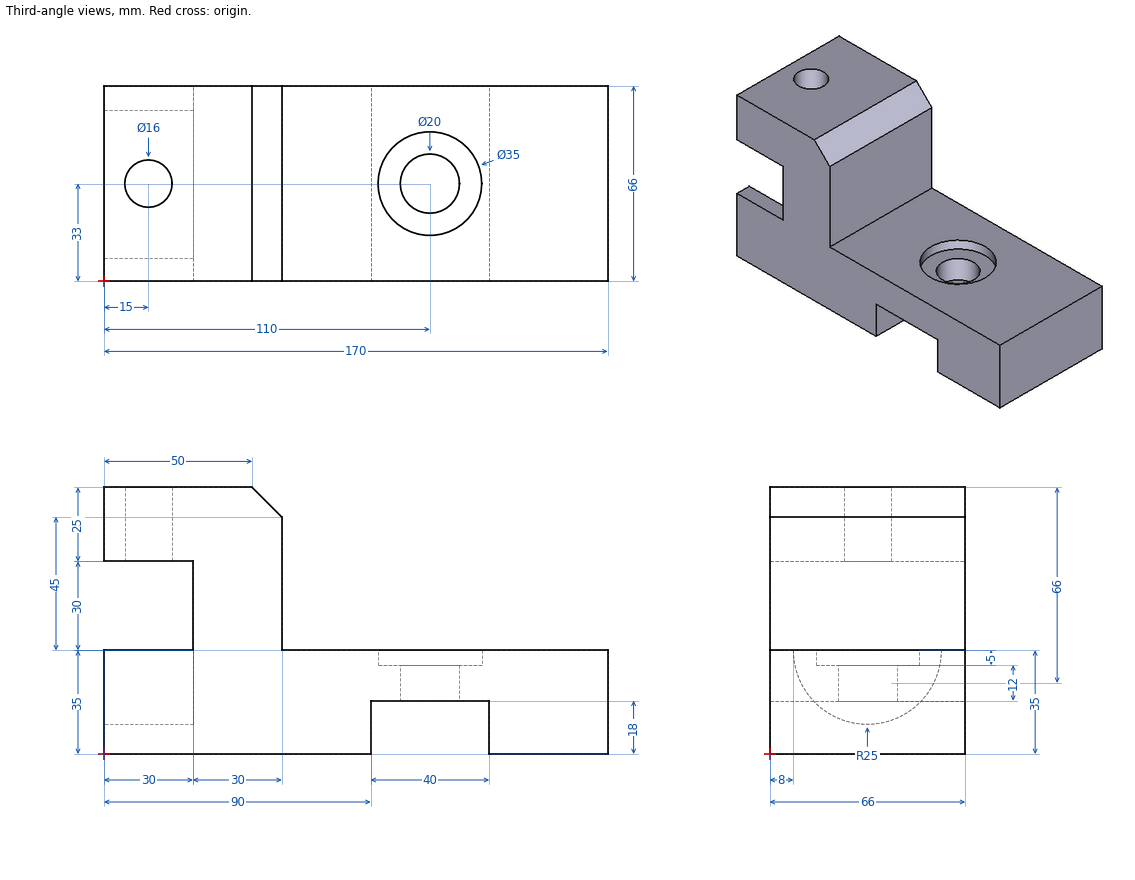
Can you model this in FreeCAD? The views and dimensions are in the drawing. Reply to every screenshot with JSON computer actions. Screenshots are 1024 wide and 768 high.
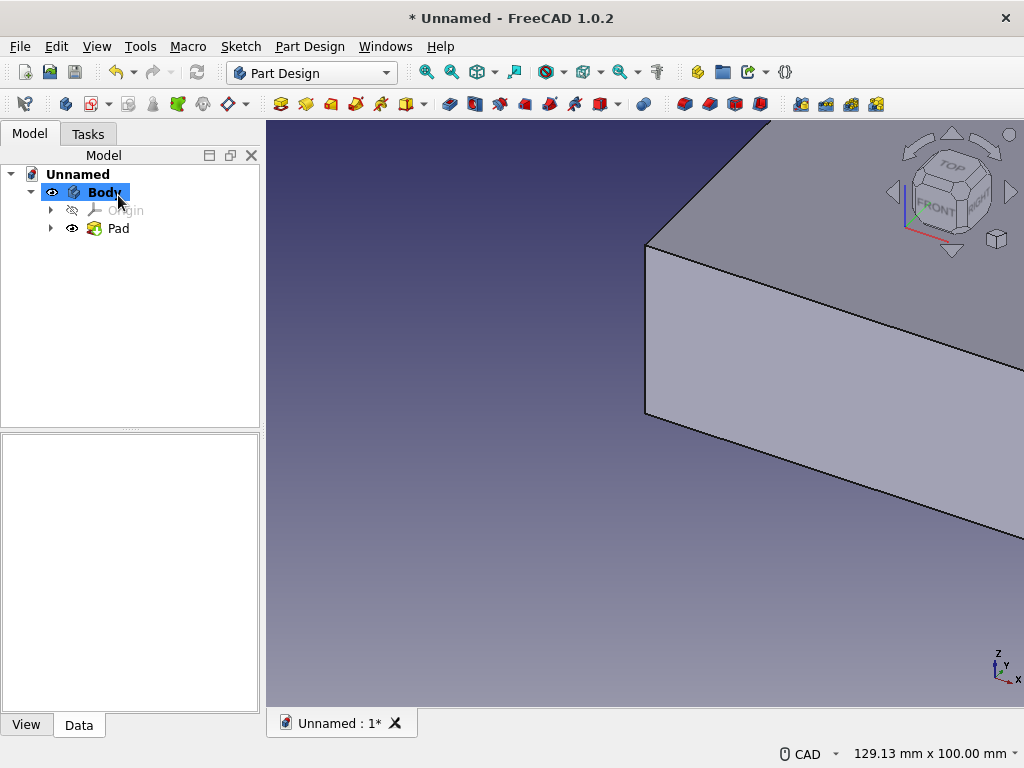
{"action": "key", "text": "v f"}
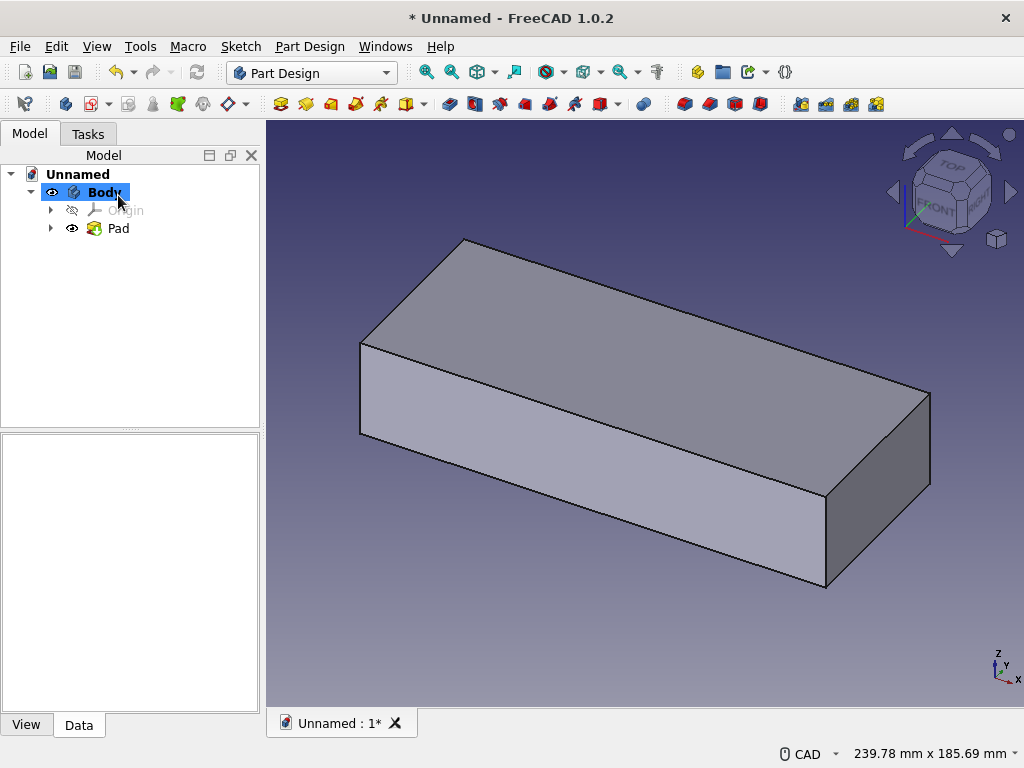
{"action": "left_click", "coordinate": [90, 104]}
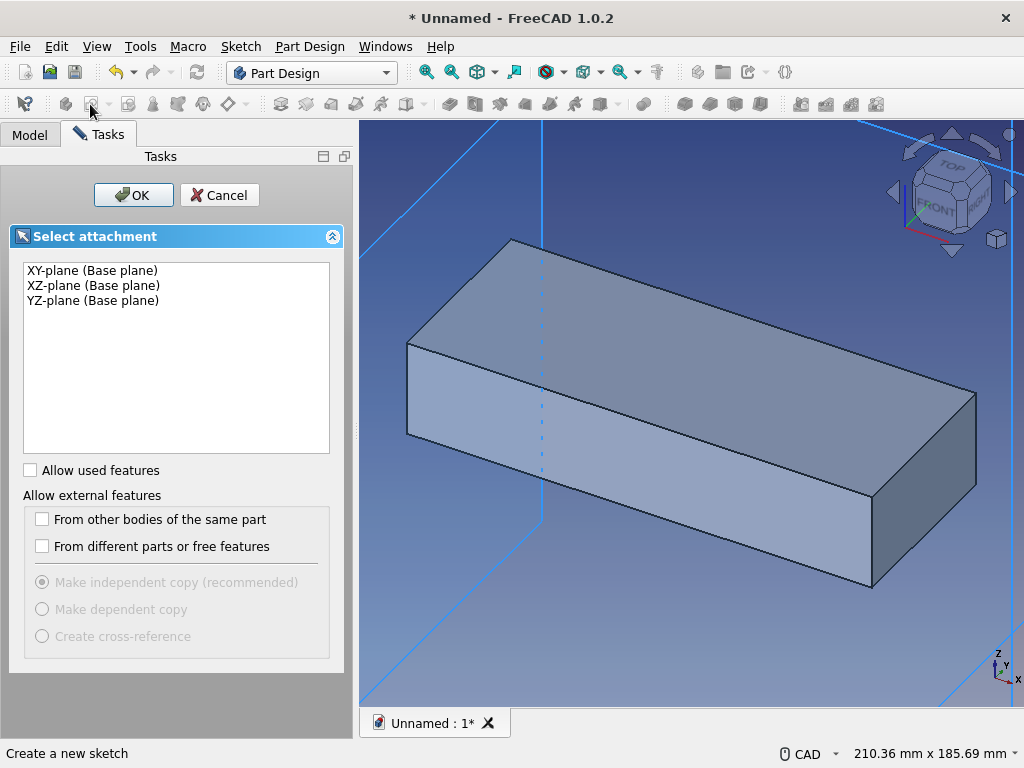
{"action": "left_click", "coordinate": [84, 286]}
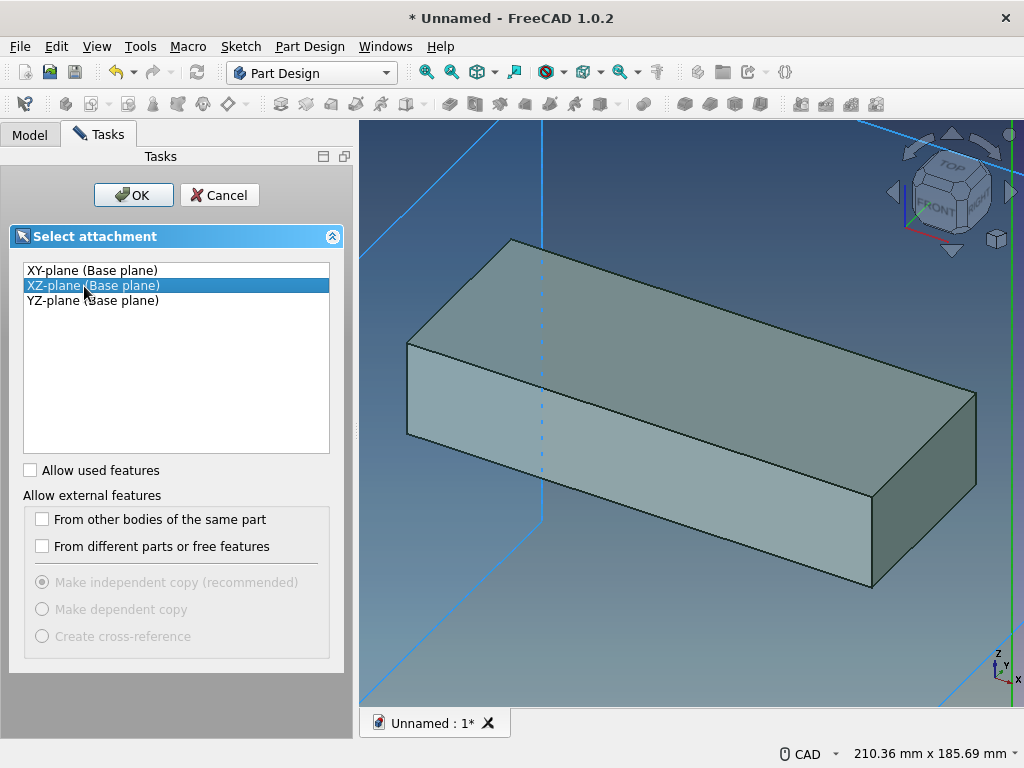
{"action": "left_click", "coordinate": [134, 195]}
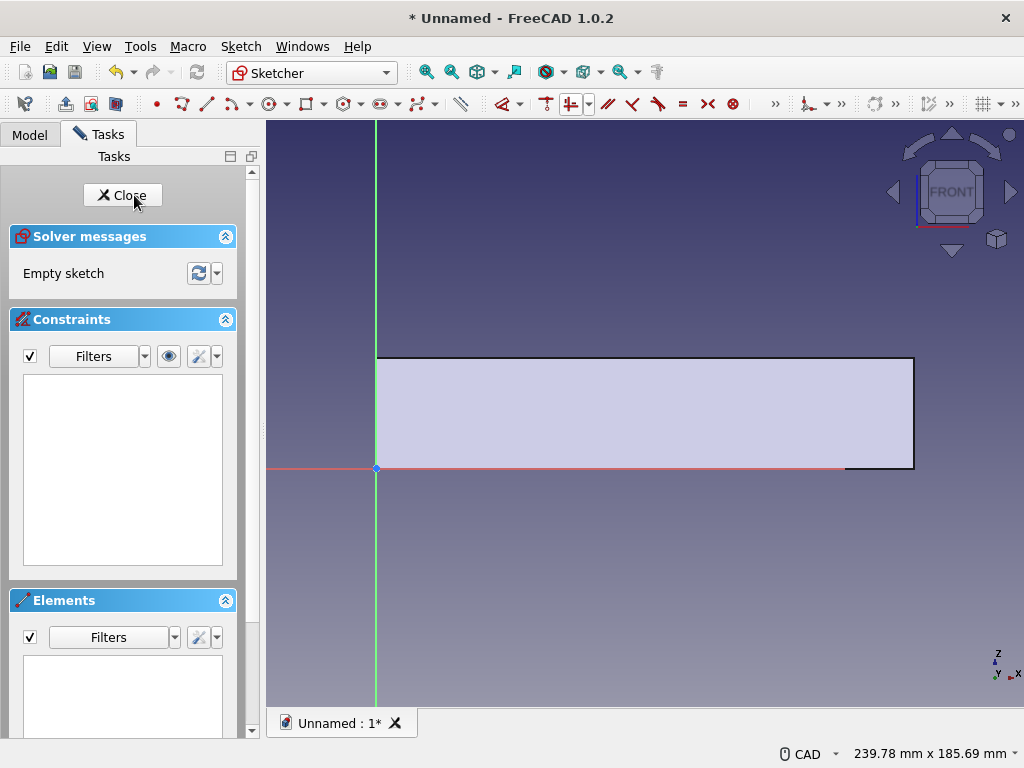
{"action": "scroll", "coordinate": [788, 452], "scroll_direction": "up", "scroll_amount": 6}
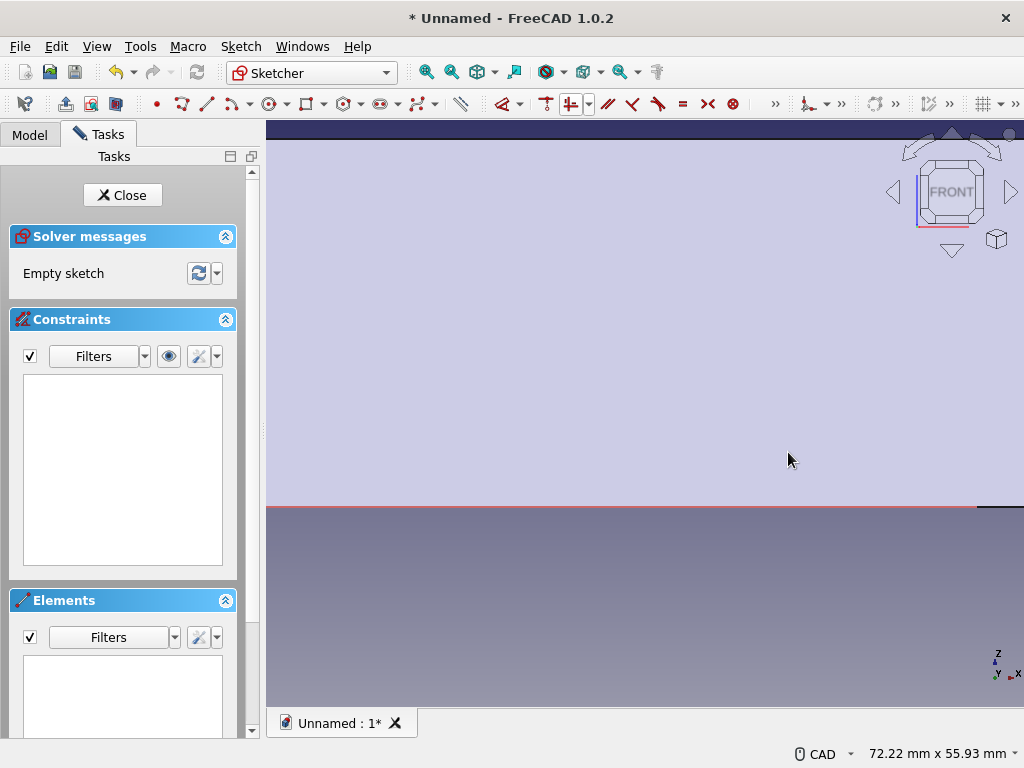
{"action": "left_click", "coordinate": [306, 104]}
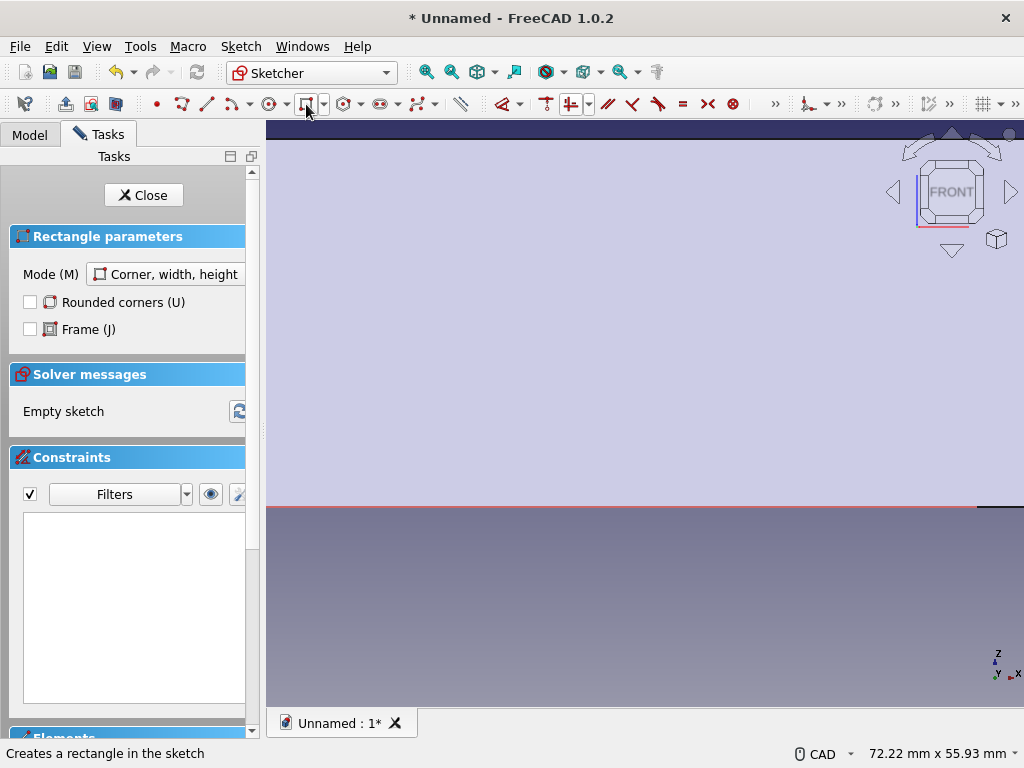
{"action": "left_click", "coordinate": [364, 318]}
{"action": "left_click", "coordinate": [784, 507]}
{"action": "key", "text": "Escape"}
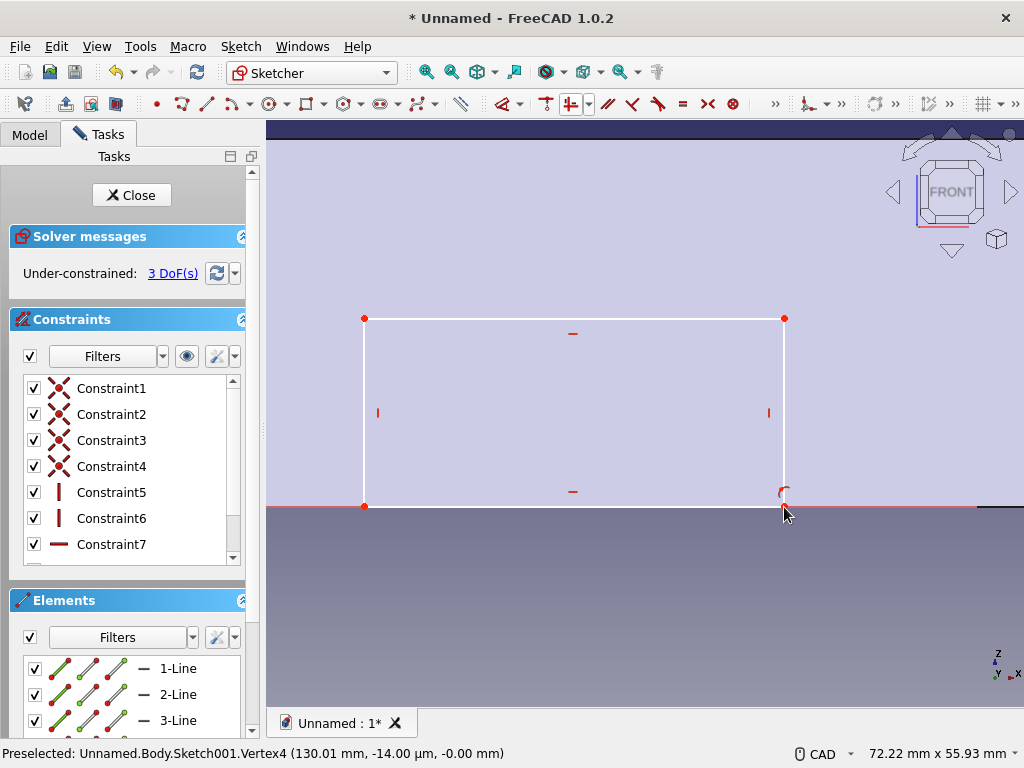
{"action": "left_click", "coordinate": [364, 375]}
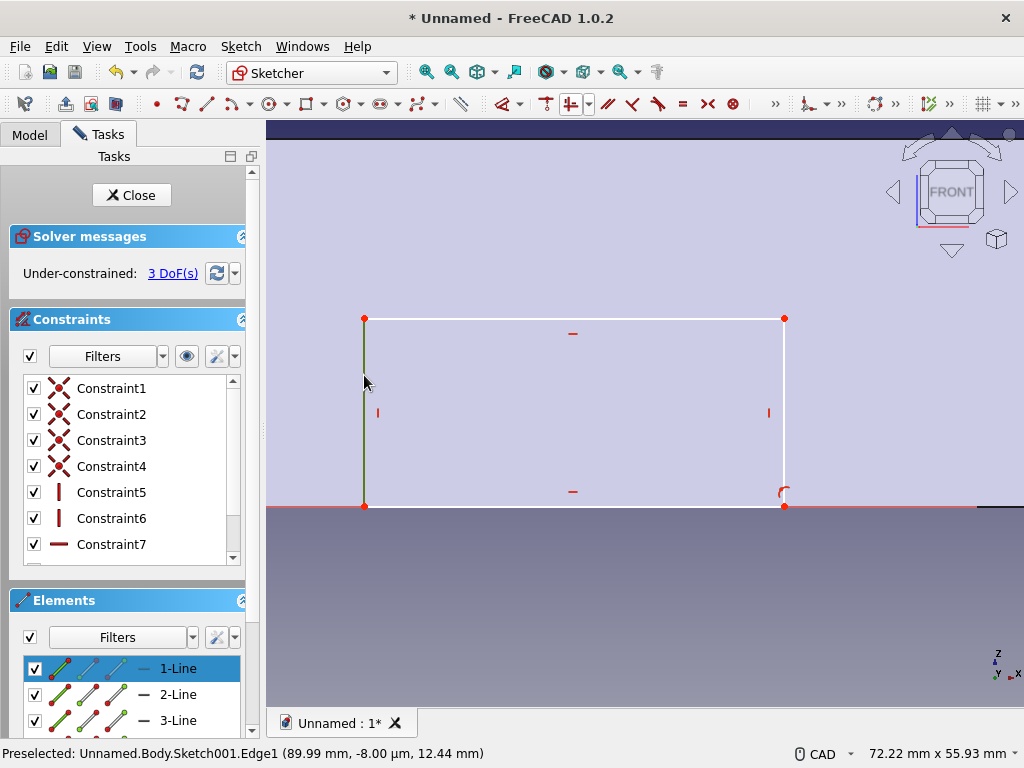
{"action": "left_click", "coordinate": [520, 104]}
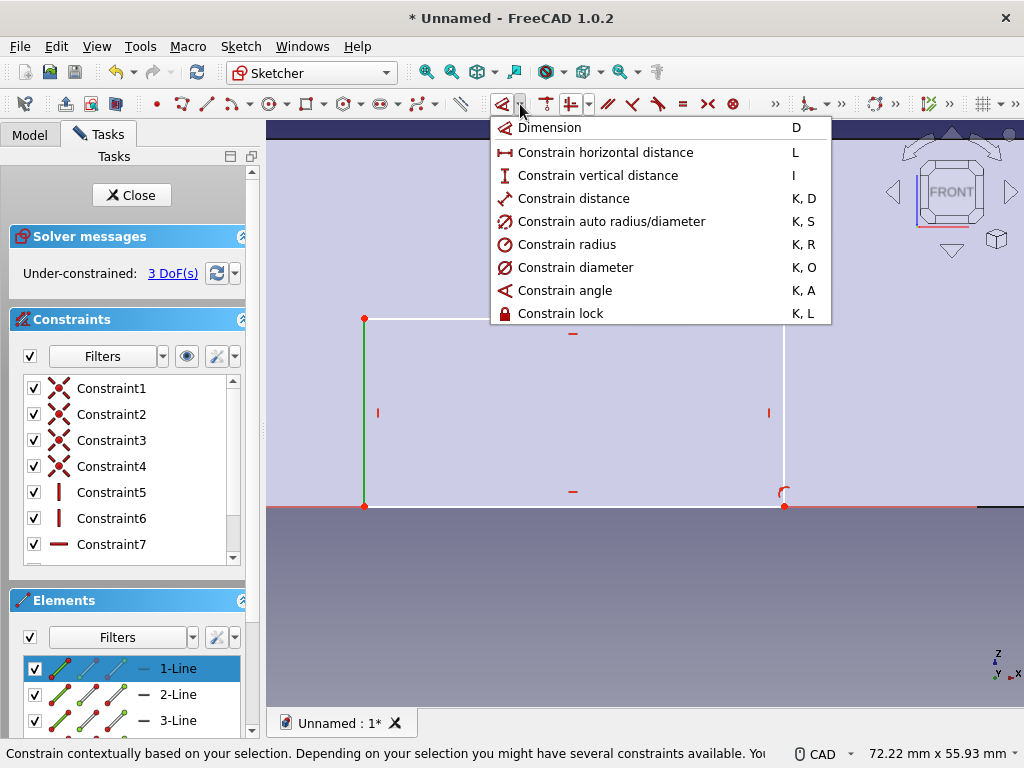
{"action": "left_click", "coordinate": [661, 176]}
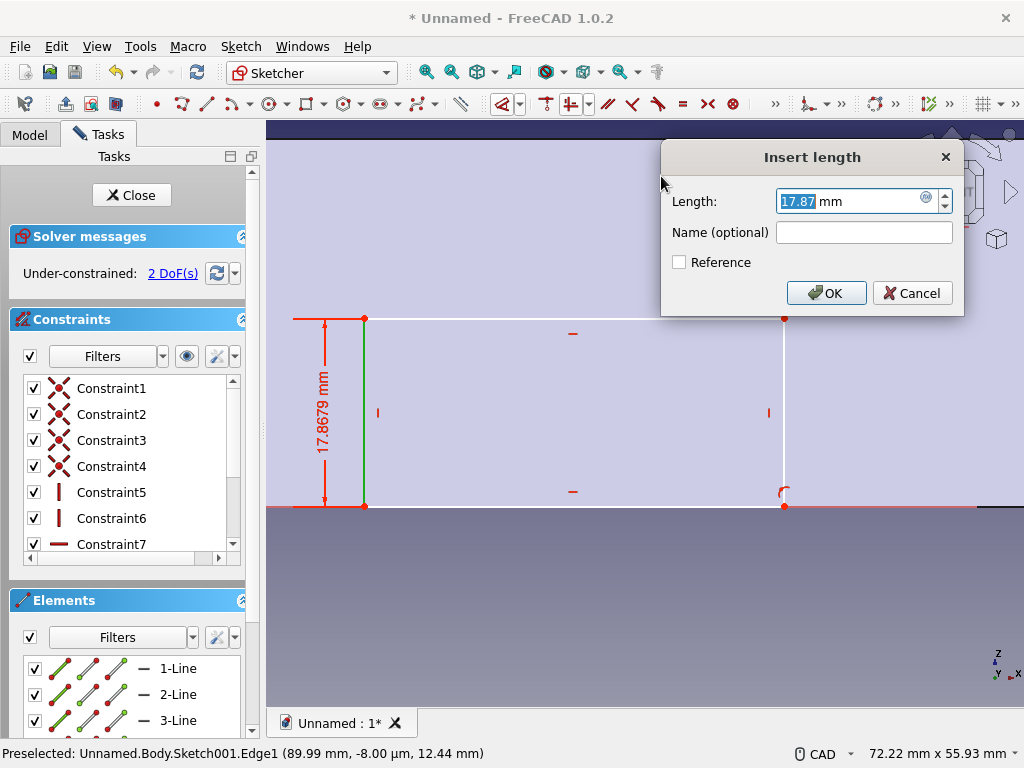
{"action": "type", "text": "18"}
{"action": "key", "text": "Return"}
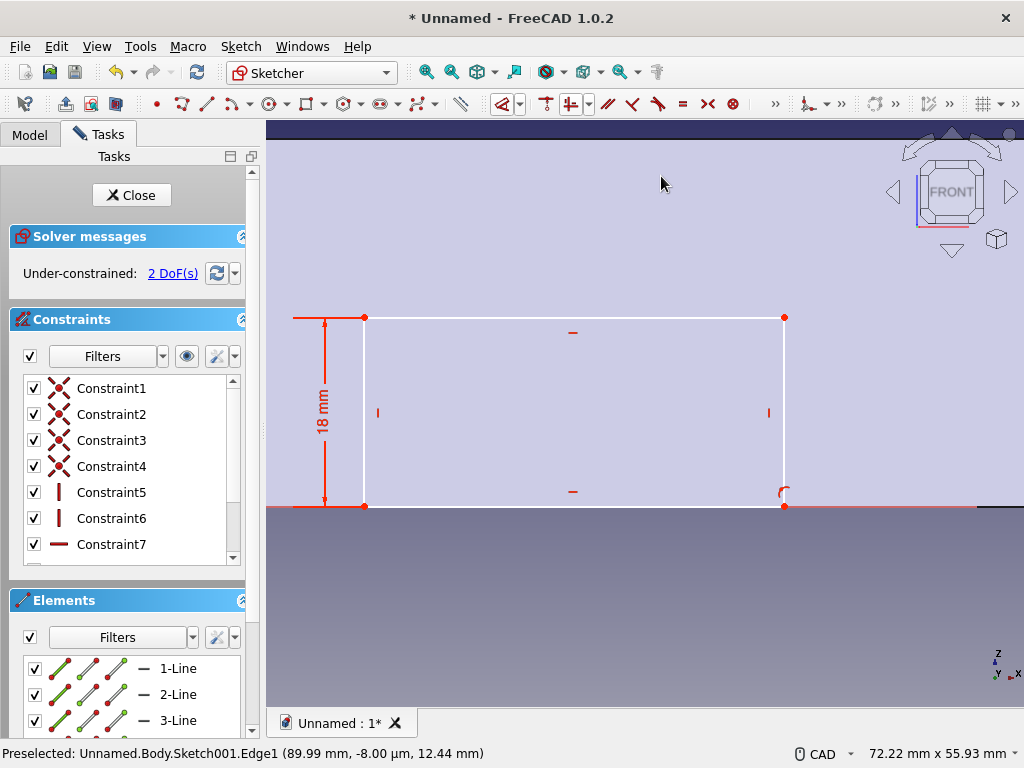
{"action": "left_click", "coordinate": [490, 507]}